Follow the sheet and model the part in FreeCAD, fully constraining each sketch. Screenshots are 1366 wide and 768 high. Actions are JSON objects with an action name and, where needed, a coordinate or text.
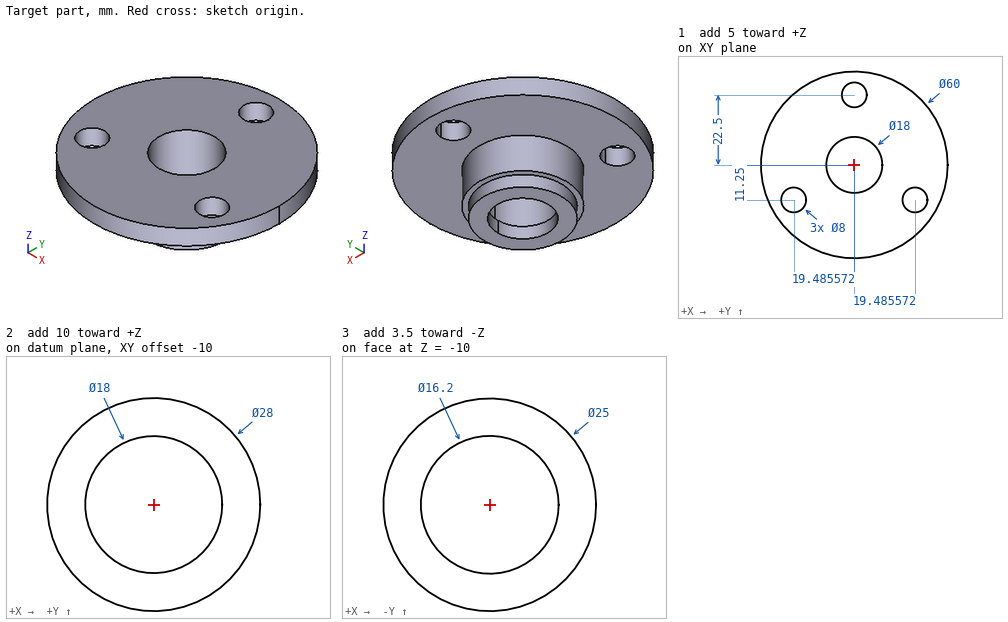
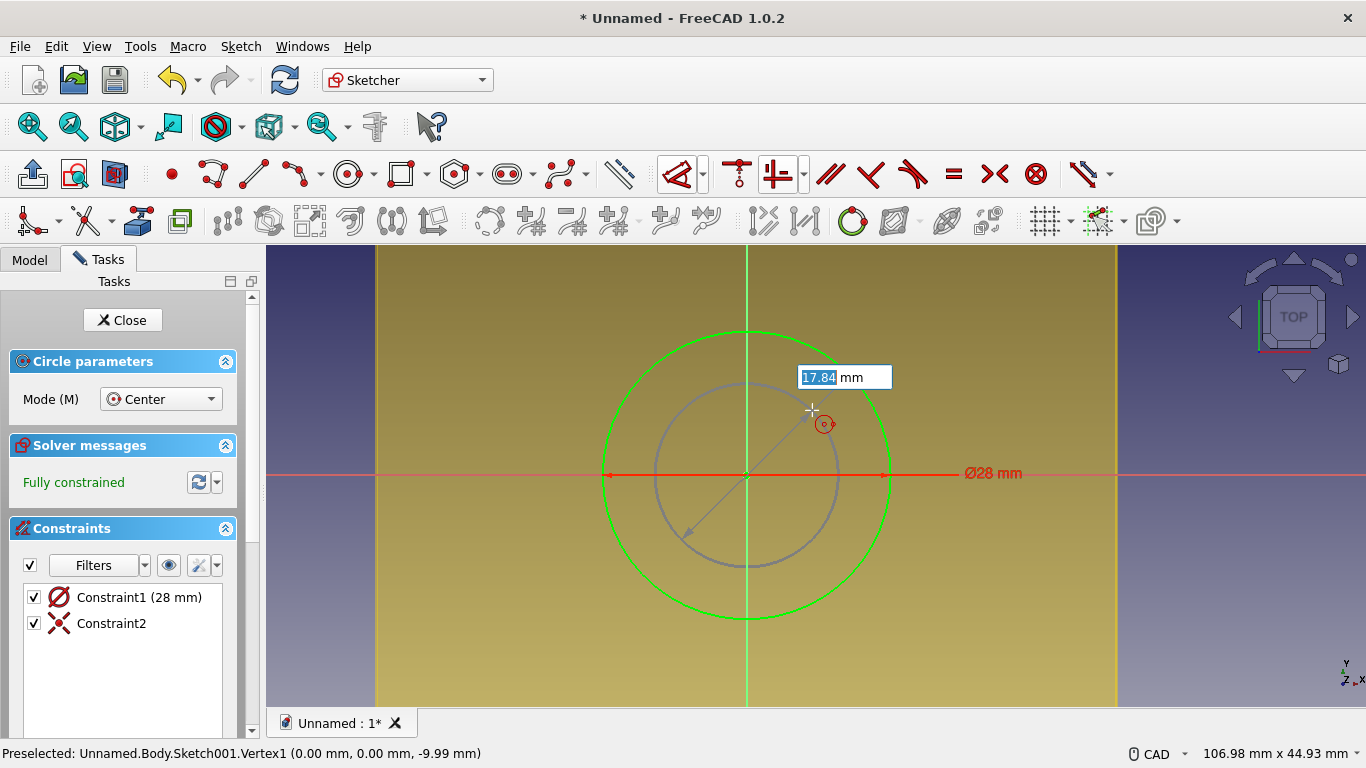
{"action": "type", "text": "18"}
{"action": "key", "text": "Return"}
{"action": "key", "text": "Escape"}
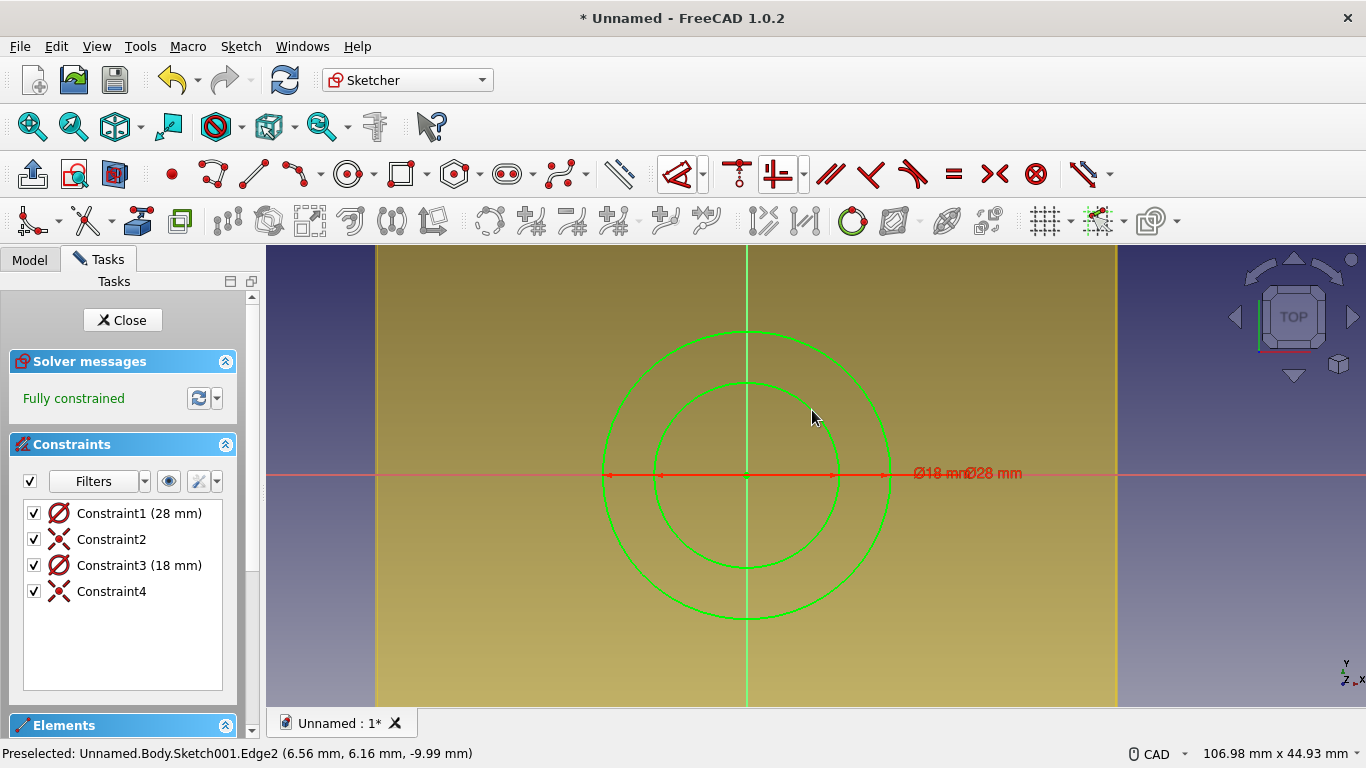
{"action": "left_click", "coordinate": [123, 320]}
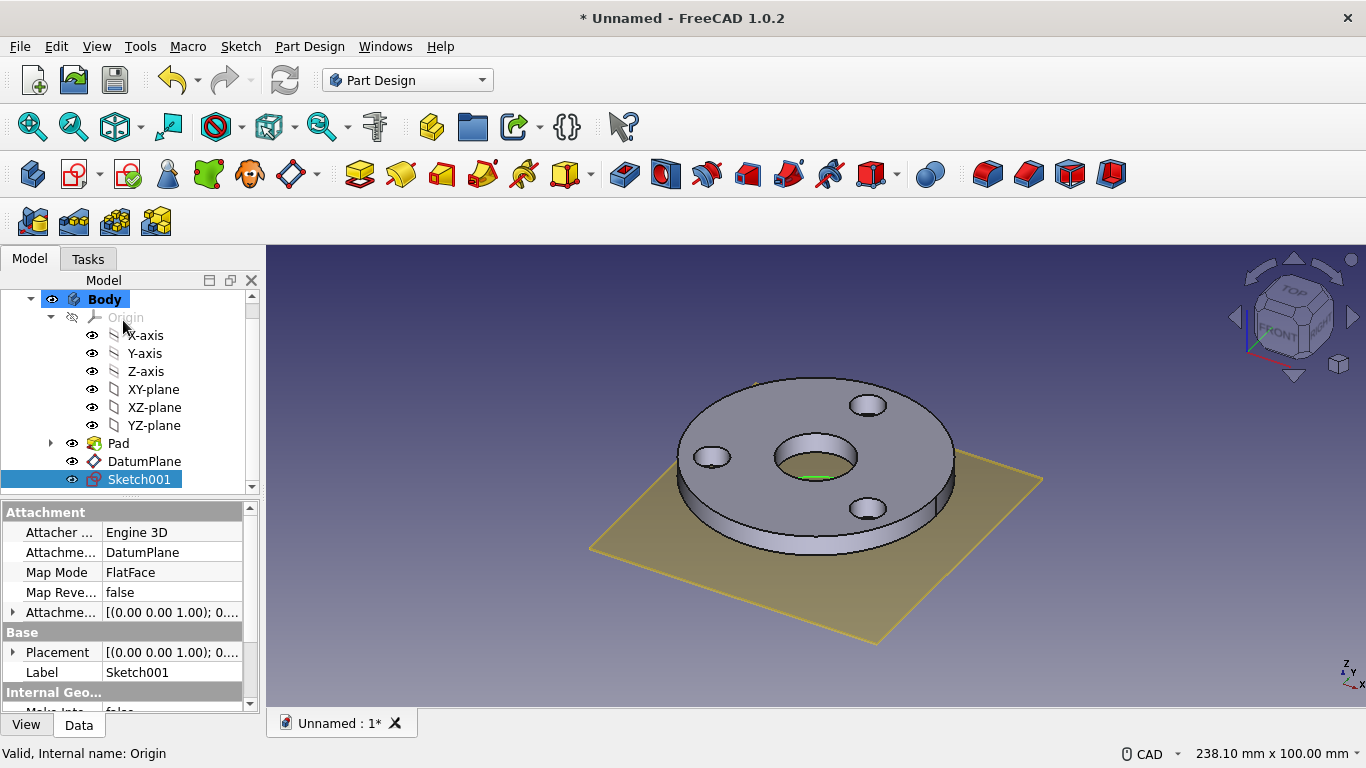
{"action": "left_click", "coordinate": [360, 174]}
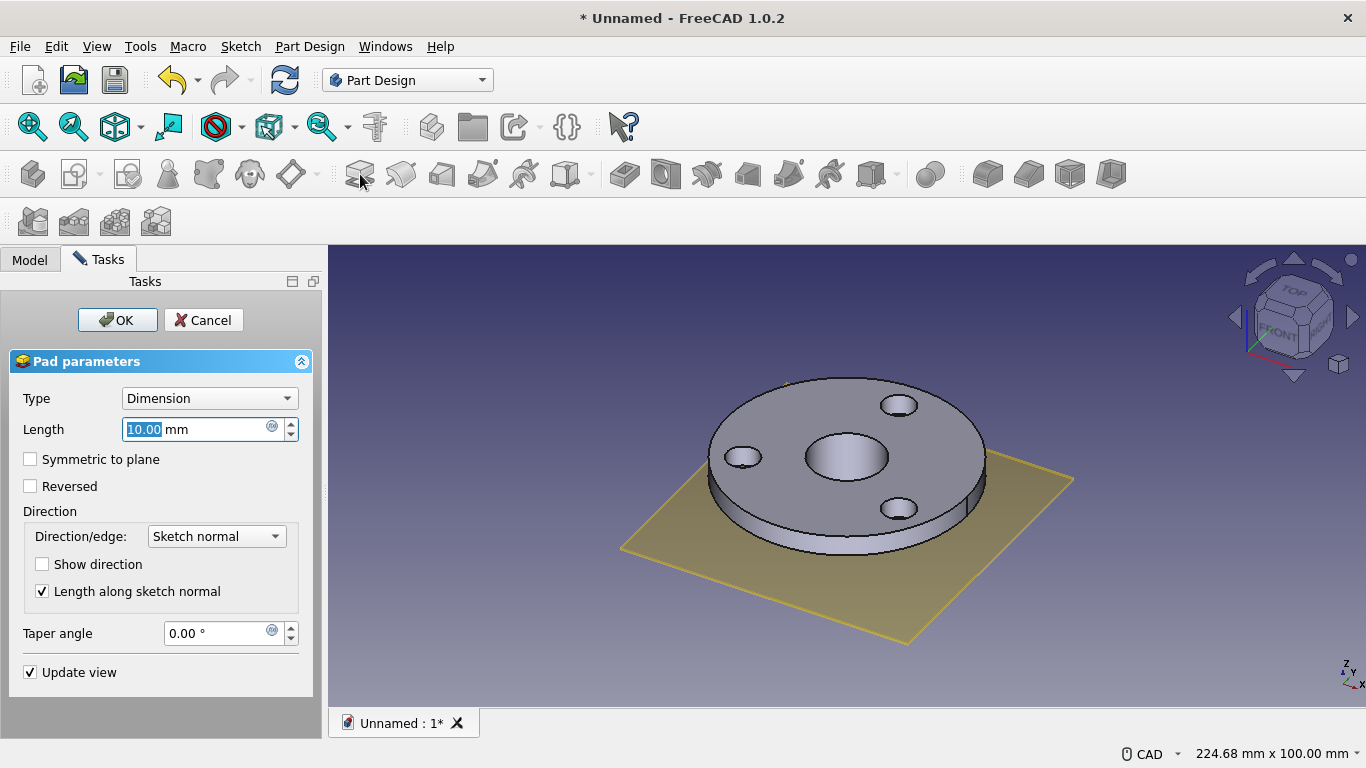
{"action": "type", "text": "10"}
{"action": "key", "text": "Tab"}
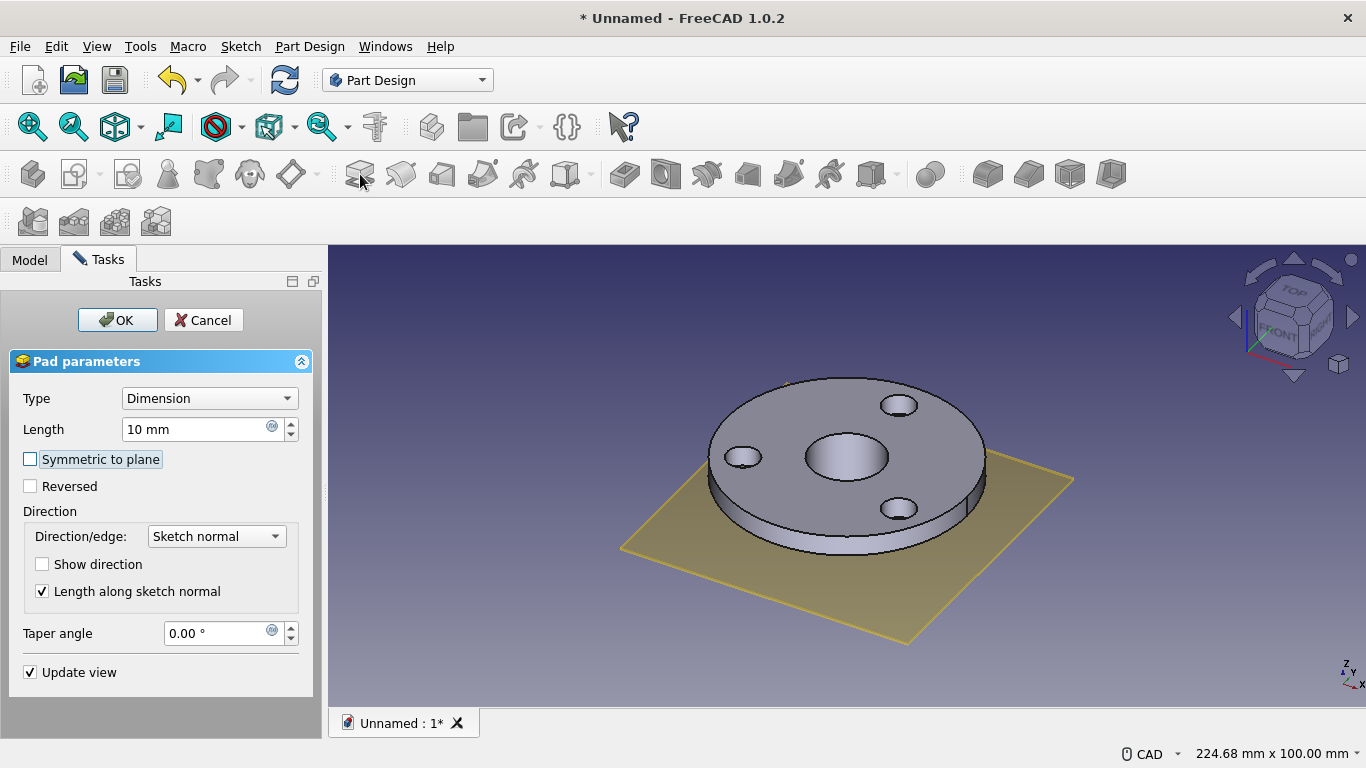
{"action": "left_click", "coordinate": [118, 320]}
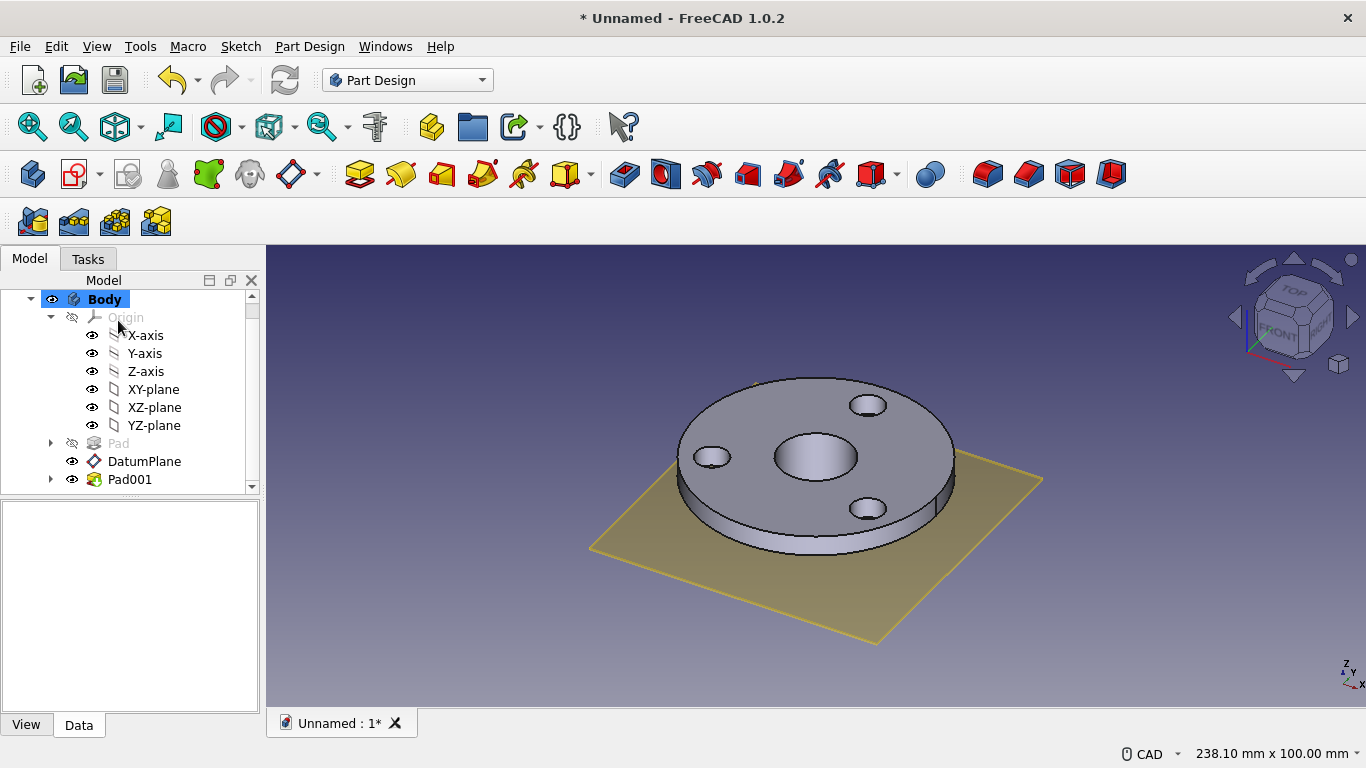
{"action": "left_click", "coordinate": [117, 461]}
{"action": "key", "text": "space"}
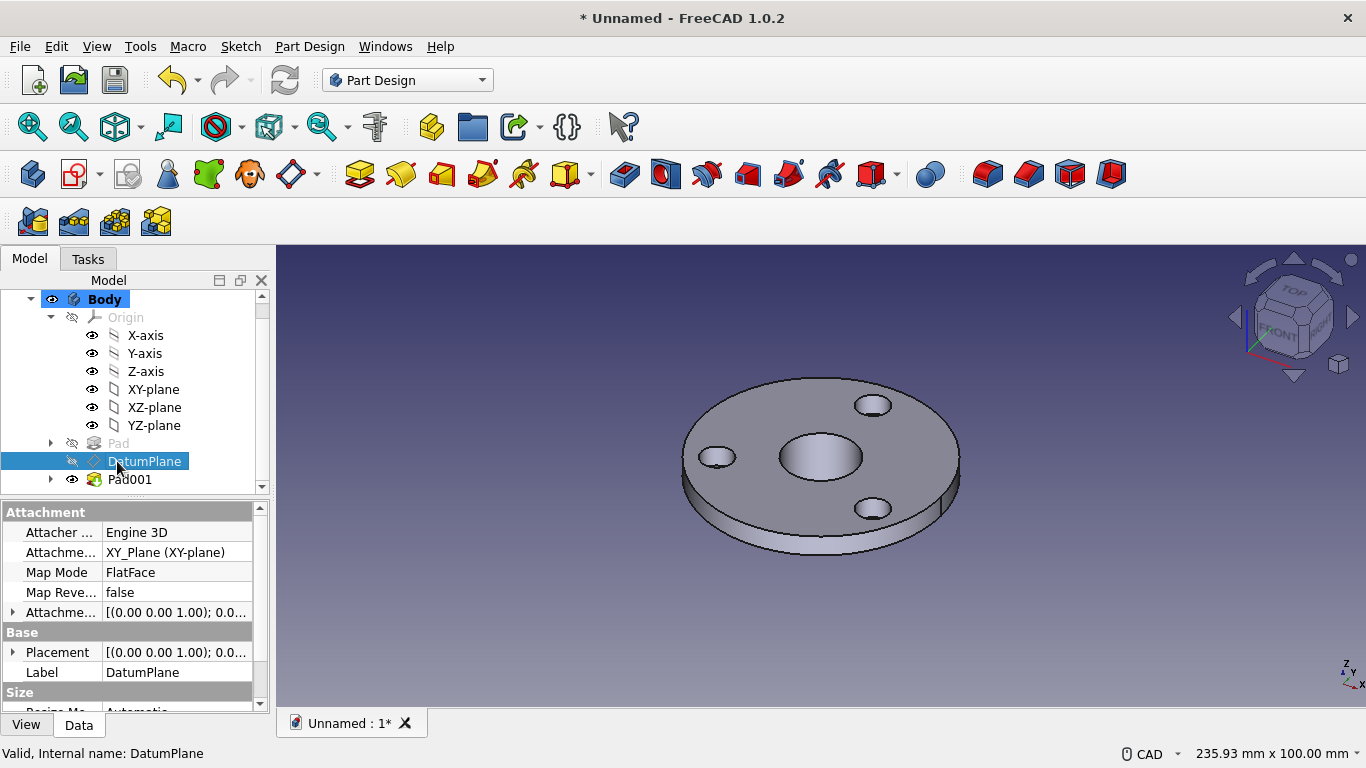
{"action": "key", "text": "5"}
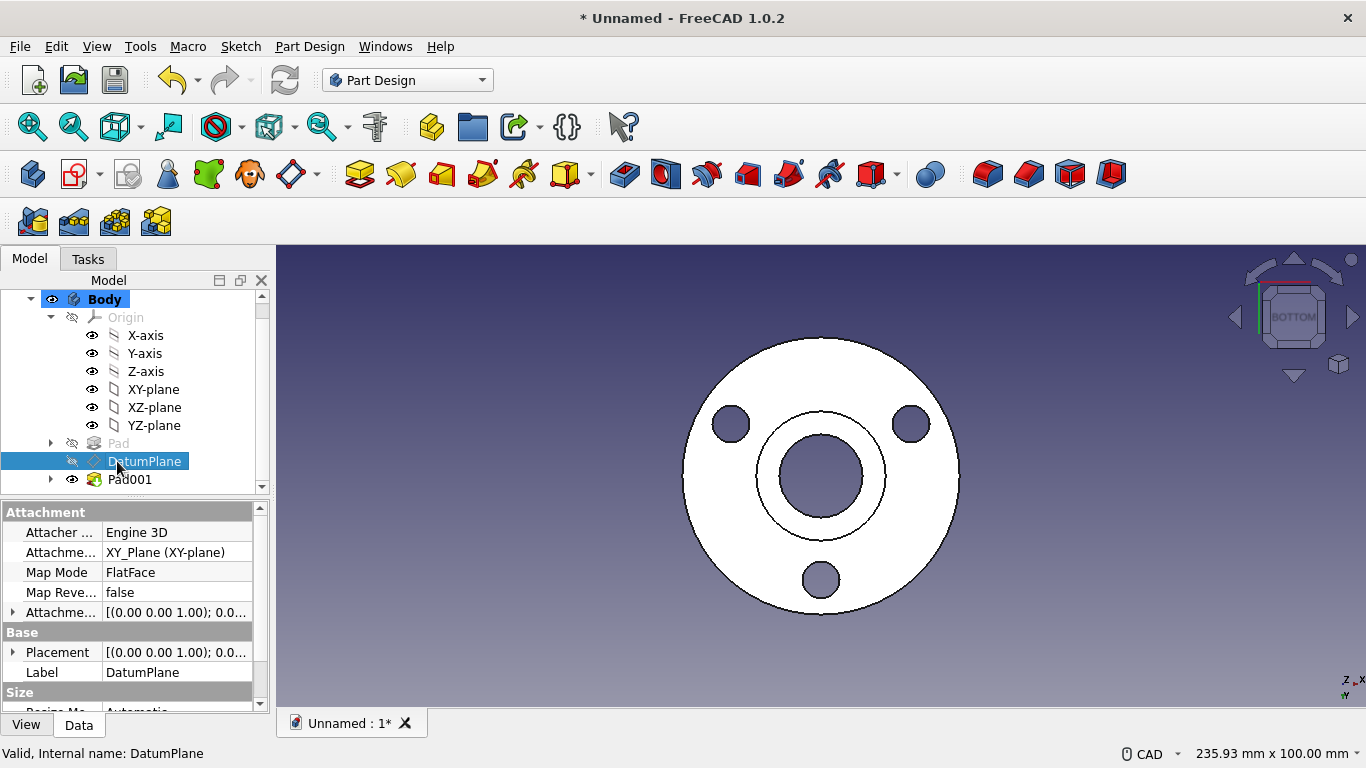
{"action": "left_click", "coordinate": [858, 512]}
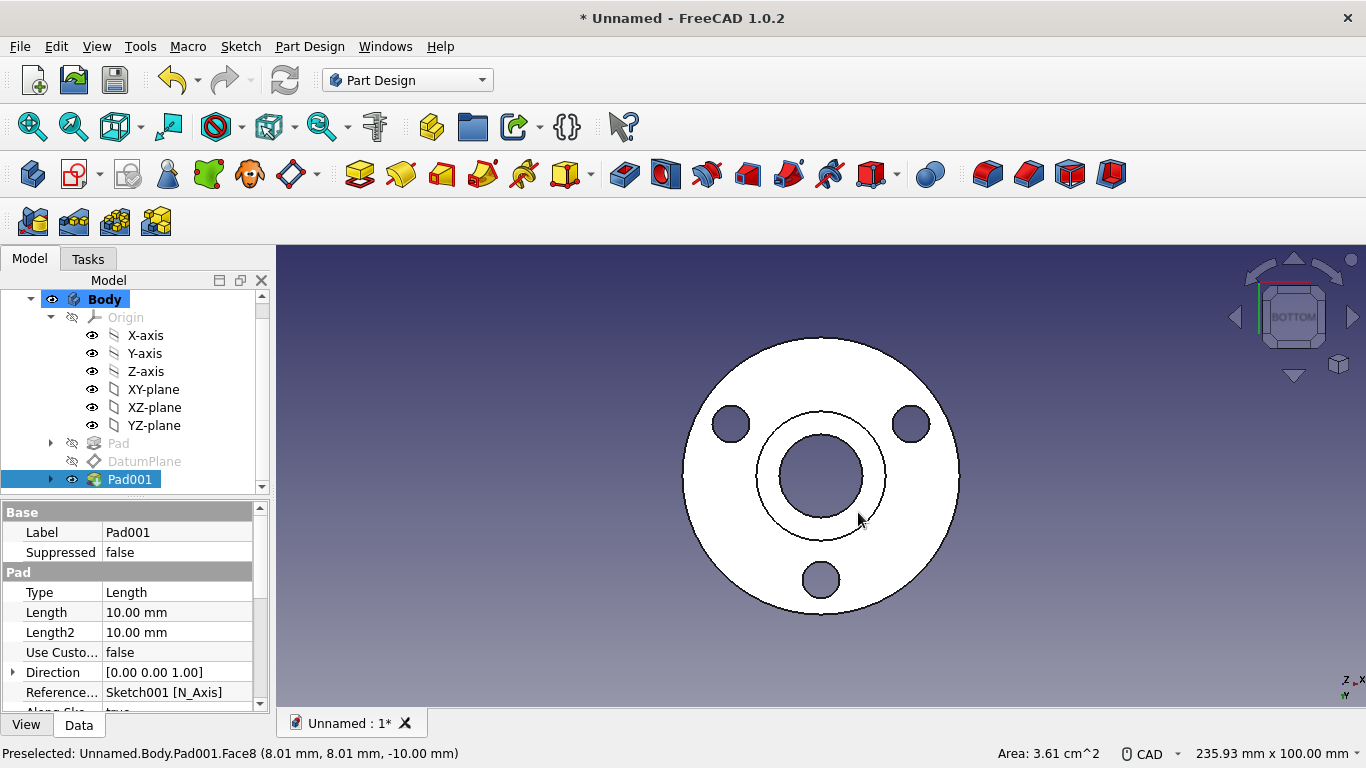
{"action": "left_click", "coordinate": [74, 174]}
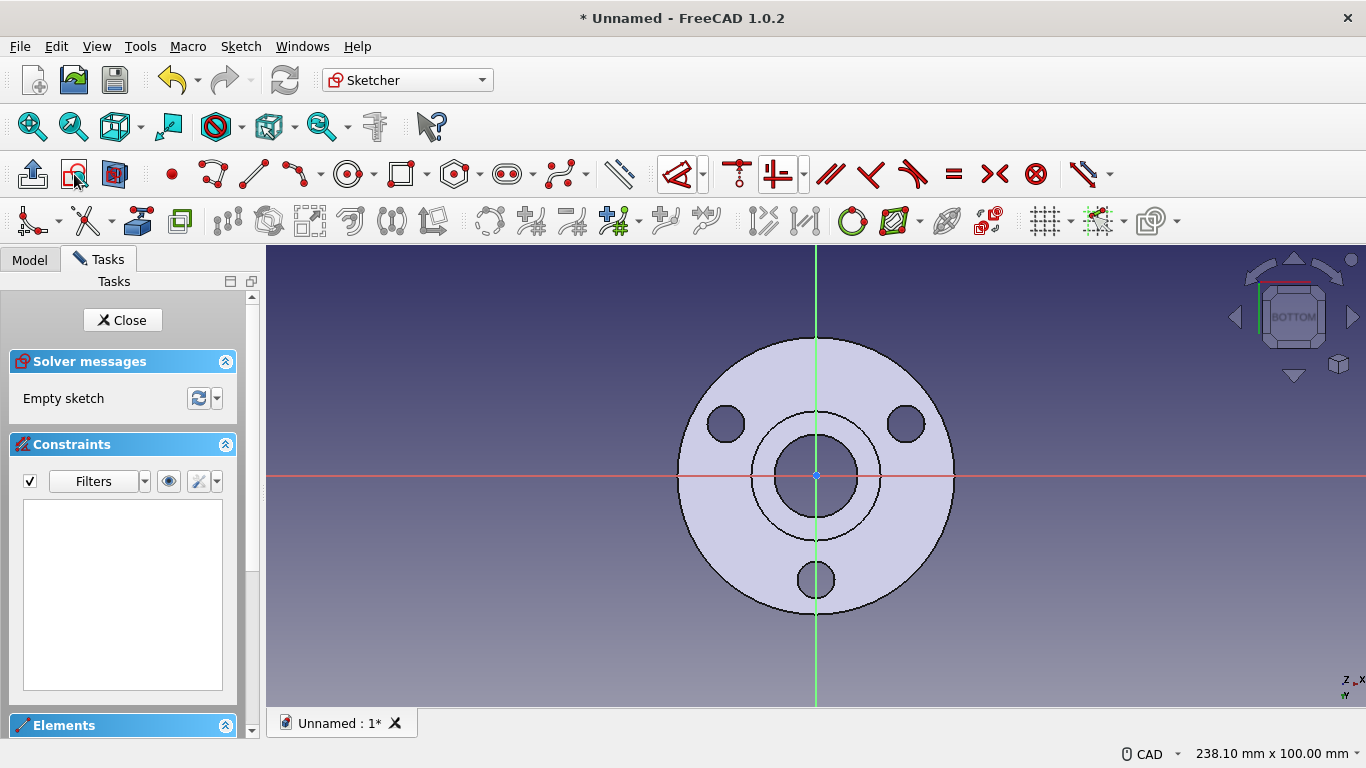
{"action": "scroll", "coordinate": [856, 476], "scroll_direction": "up", "scroll_amount": 5}